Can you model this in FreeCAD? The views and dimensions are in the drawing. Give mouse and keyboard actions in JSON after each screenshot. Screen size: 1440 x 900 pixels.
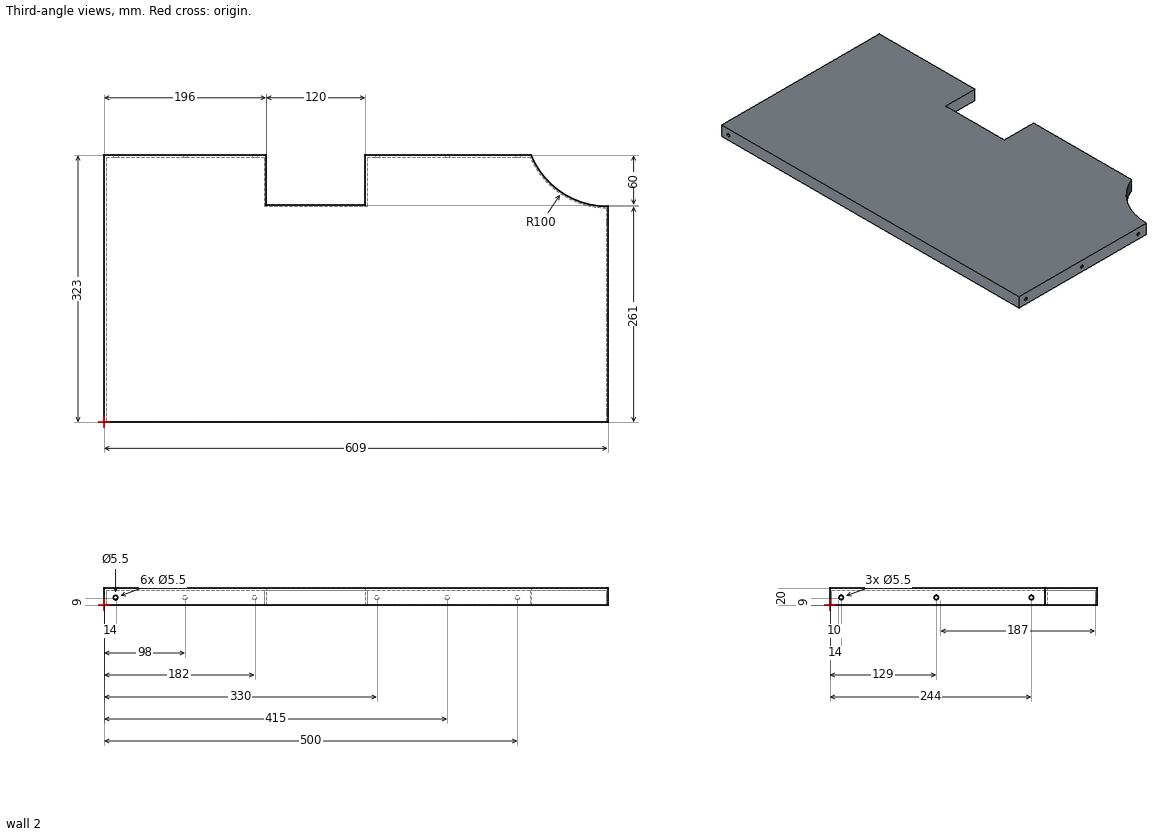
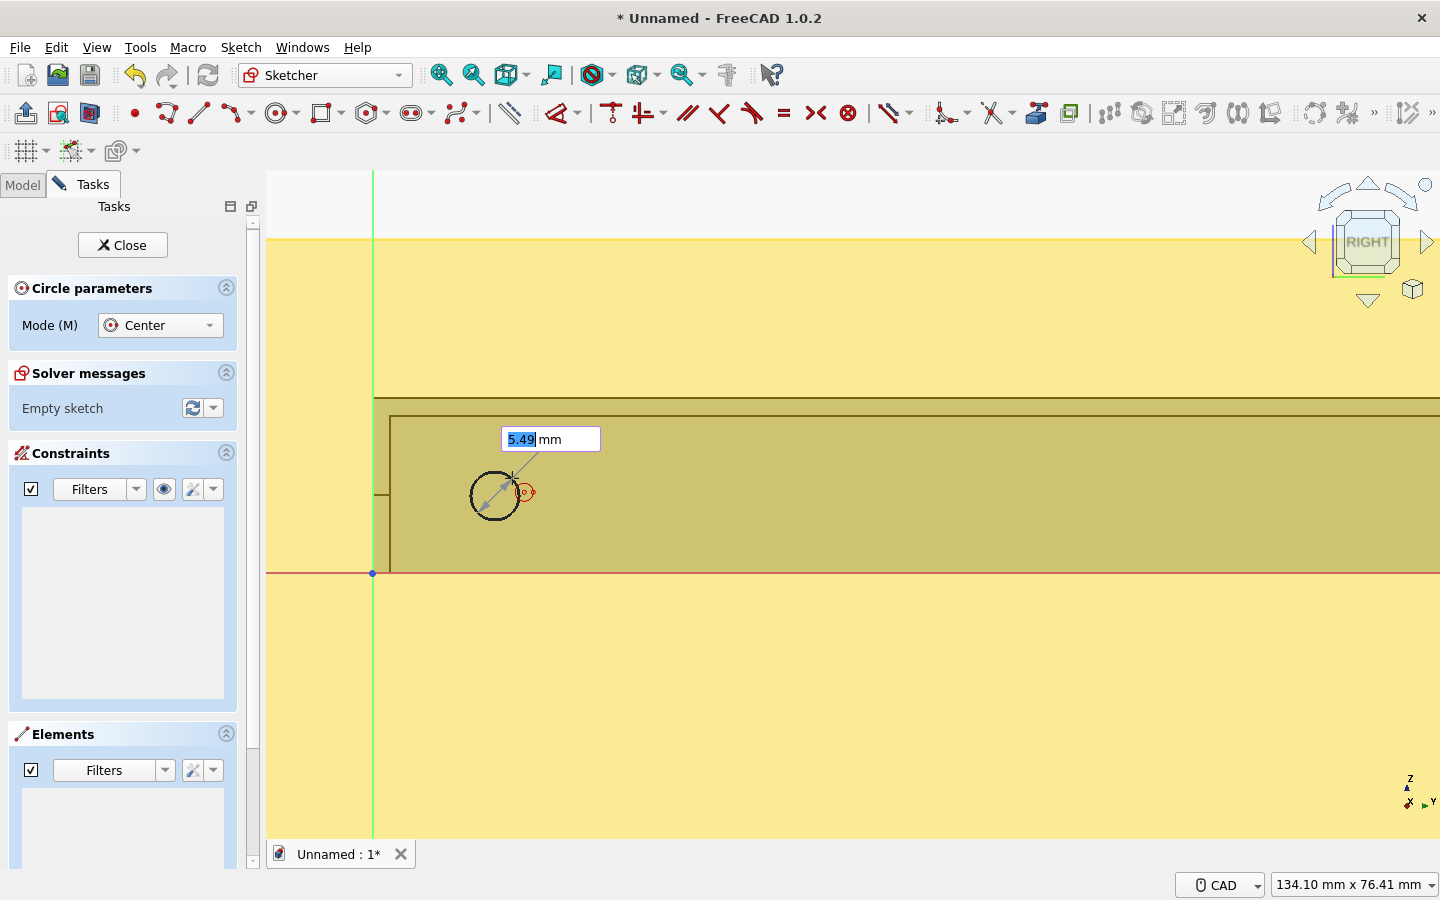
{"action": "type", "text": "5.5"}
{"action": "key", "text": "Return"}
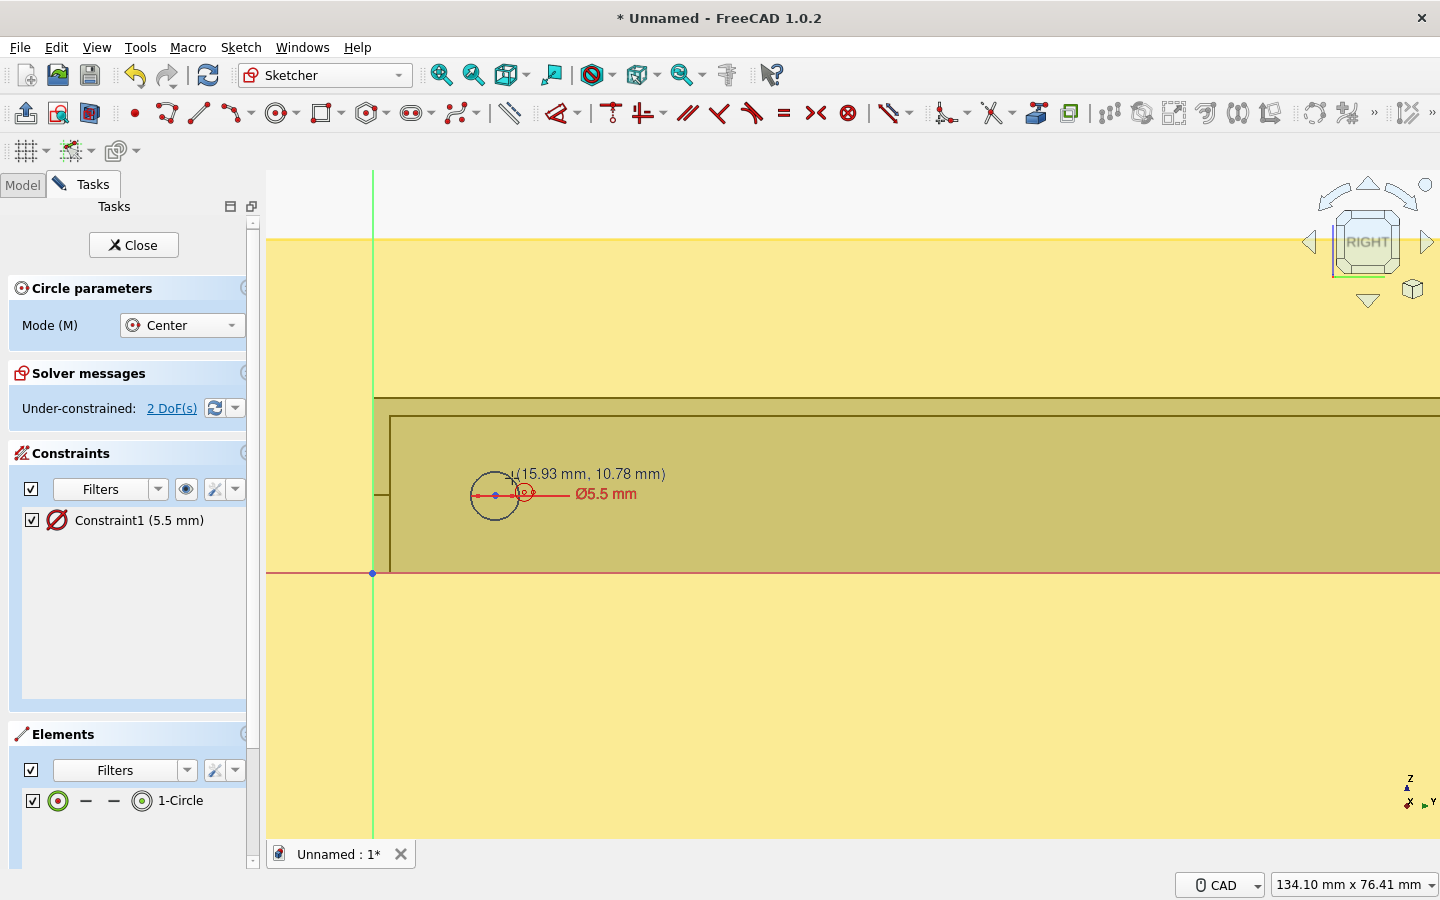
{"action": "scroll", "coordinate": [497, 497], "scroll_direction": "down", "scroll_amount": 6}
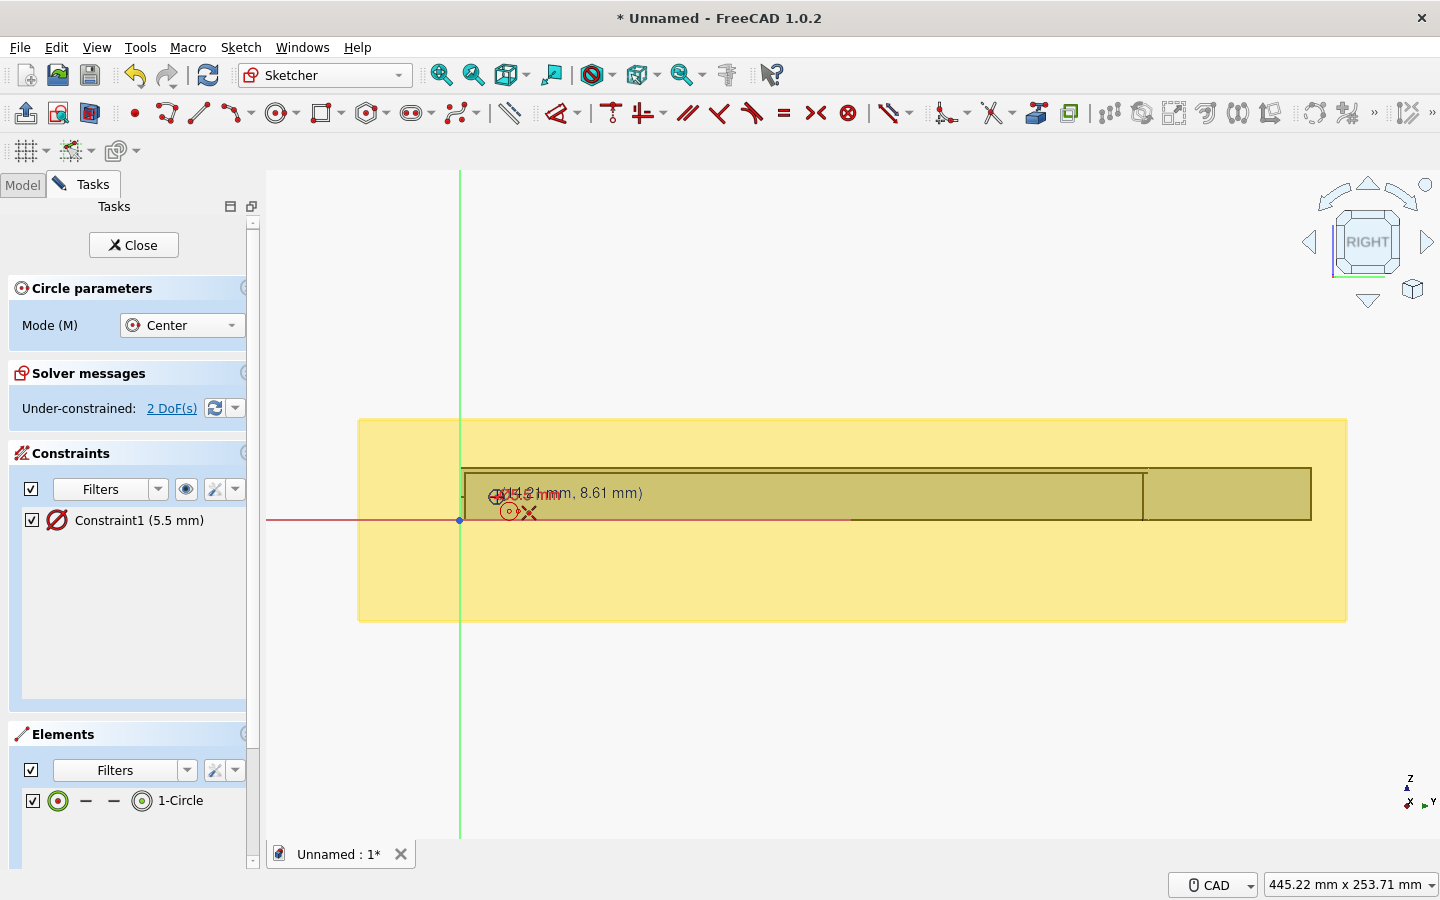
{"action": "scroll", "coordinate": [800, 497], "scroll_direction": "up", "scroll_amount": 6}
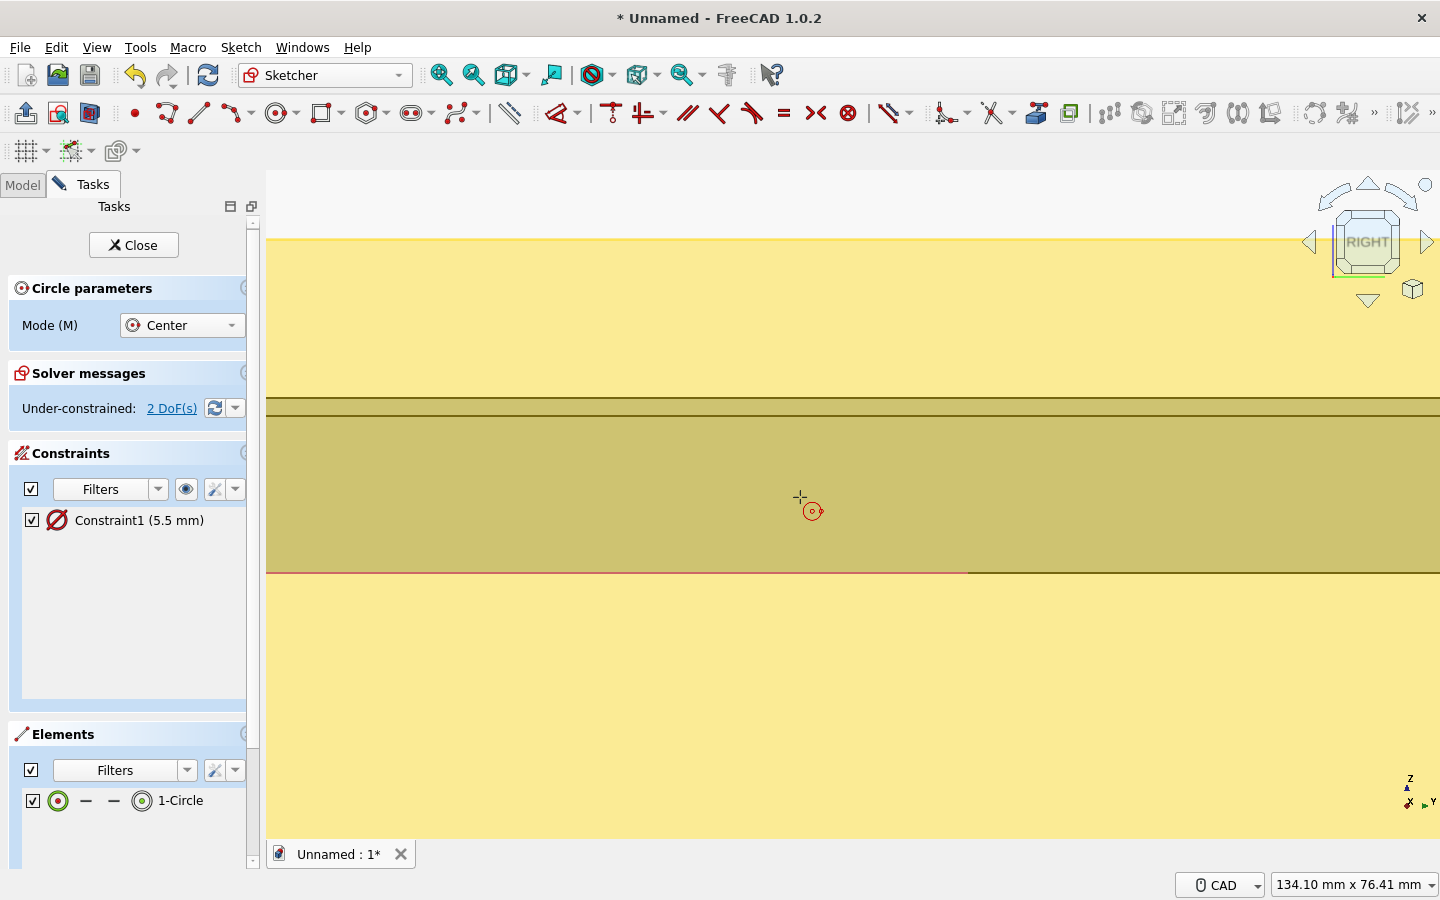
{"action": "left_click", "coordinate": [798, 495]}
{"action": "mouse_move", "coordinate": [815, 478]}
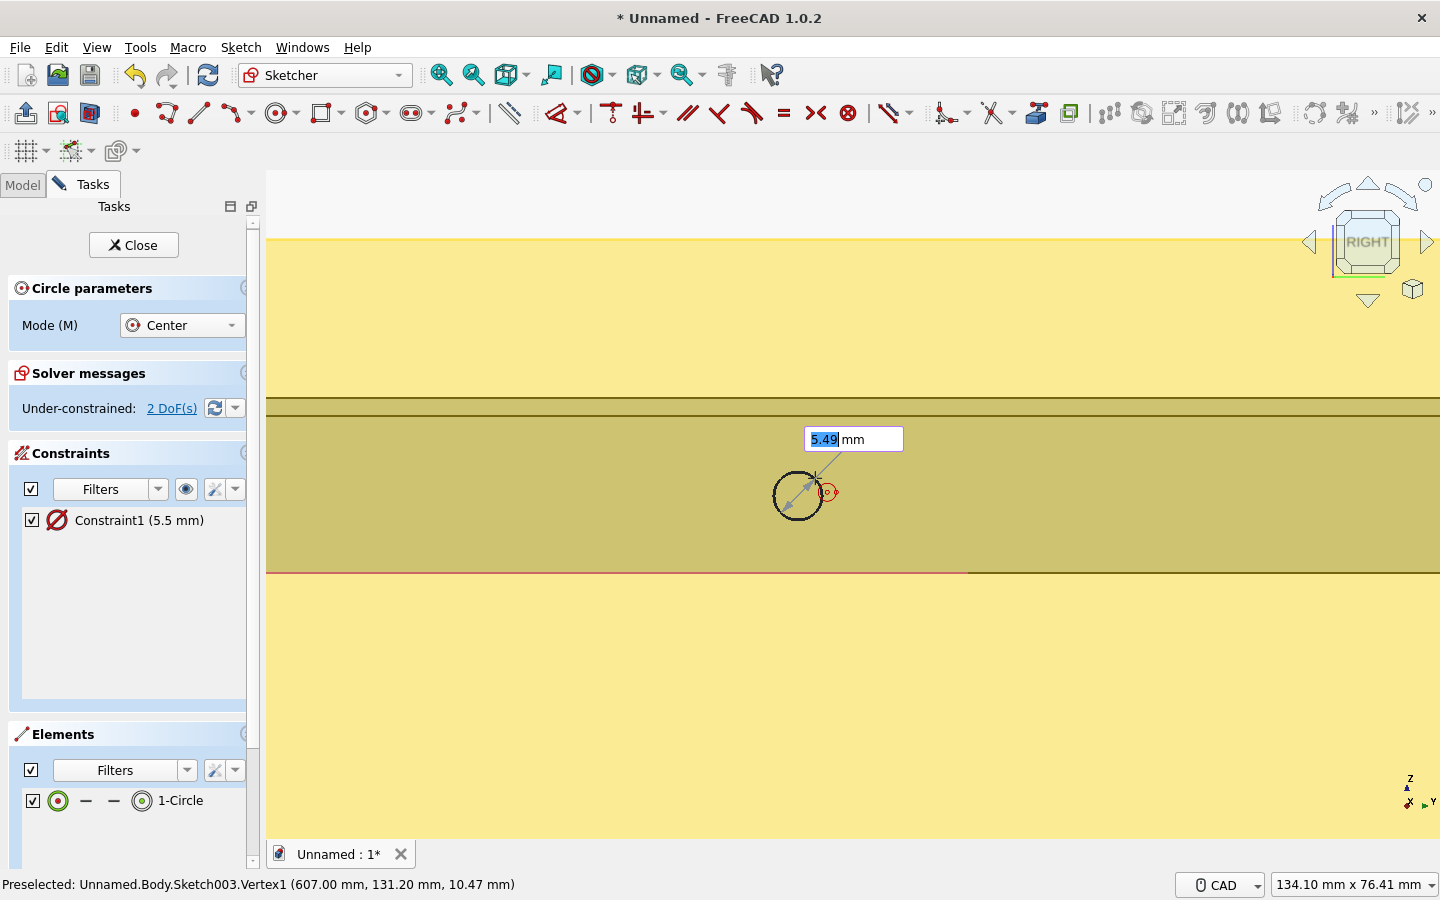
{"action": "type", "text": "5.5"}
{"action": "key", "text": "Return"}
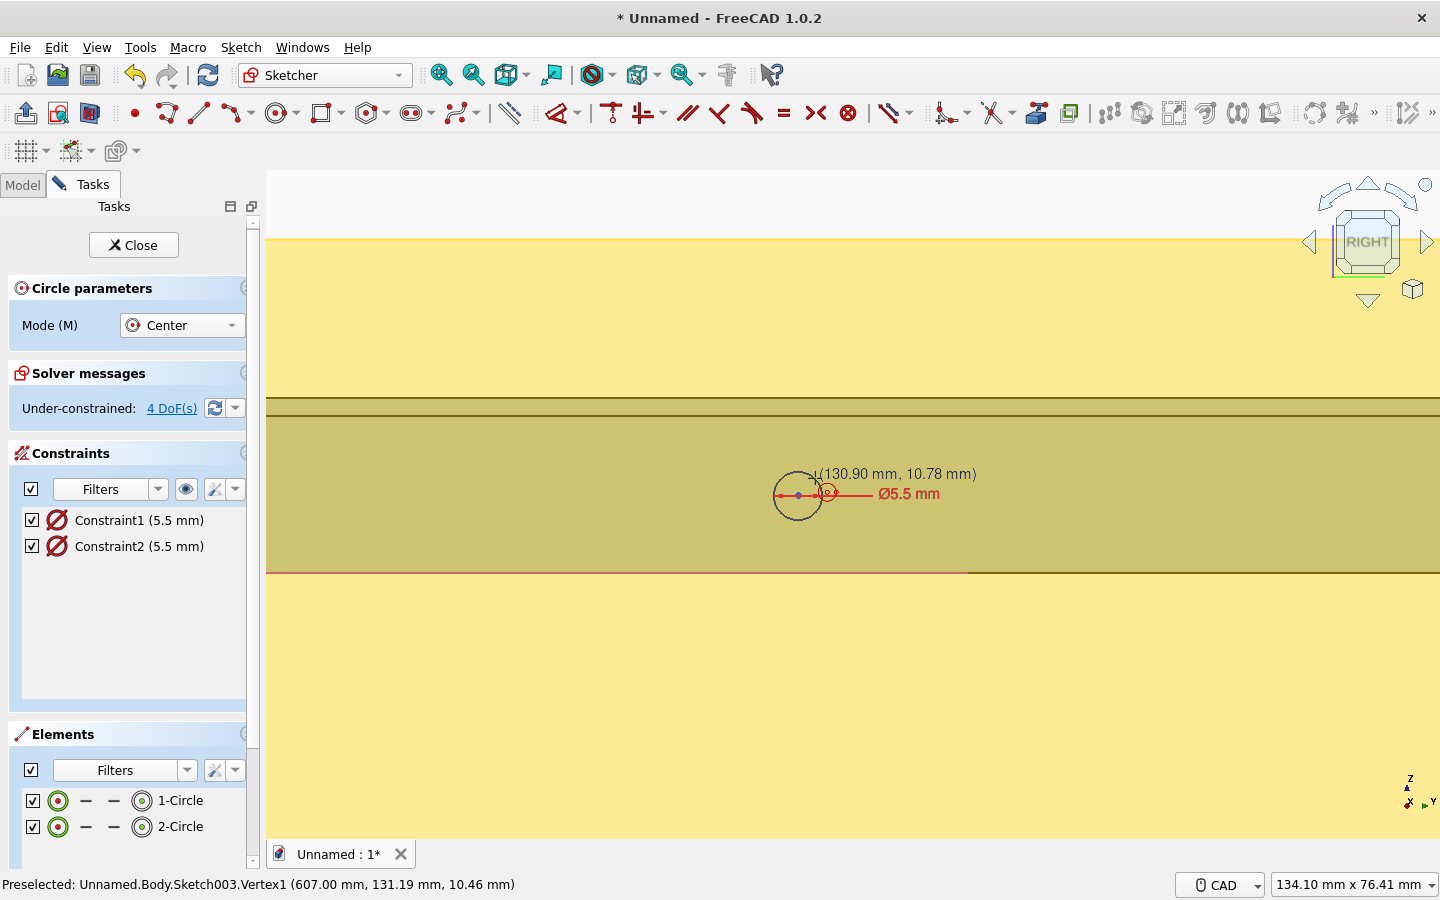
{"action": "scroll", "coordinate": [800, 497], "scroll_direction": "down", "scroll_amount": 6}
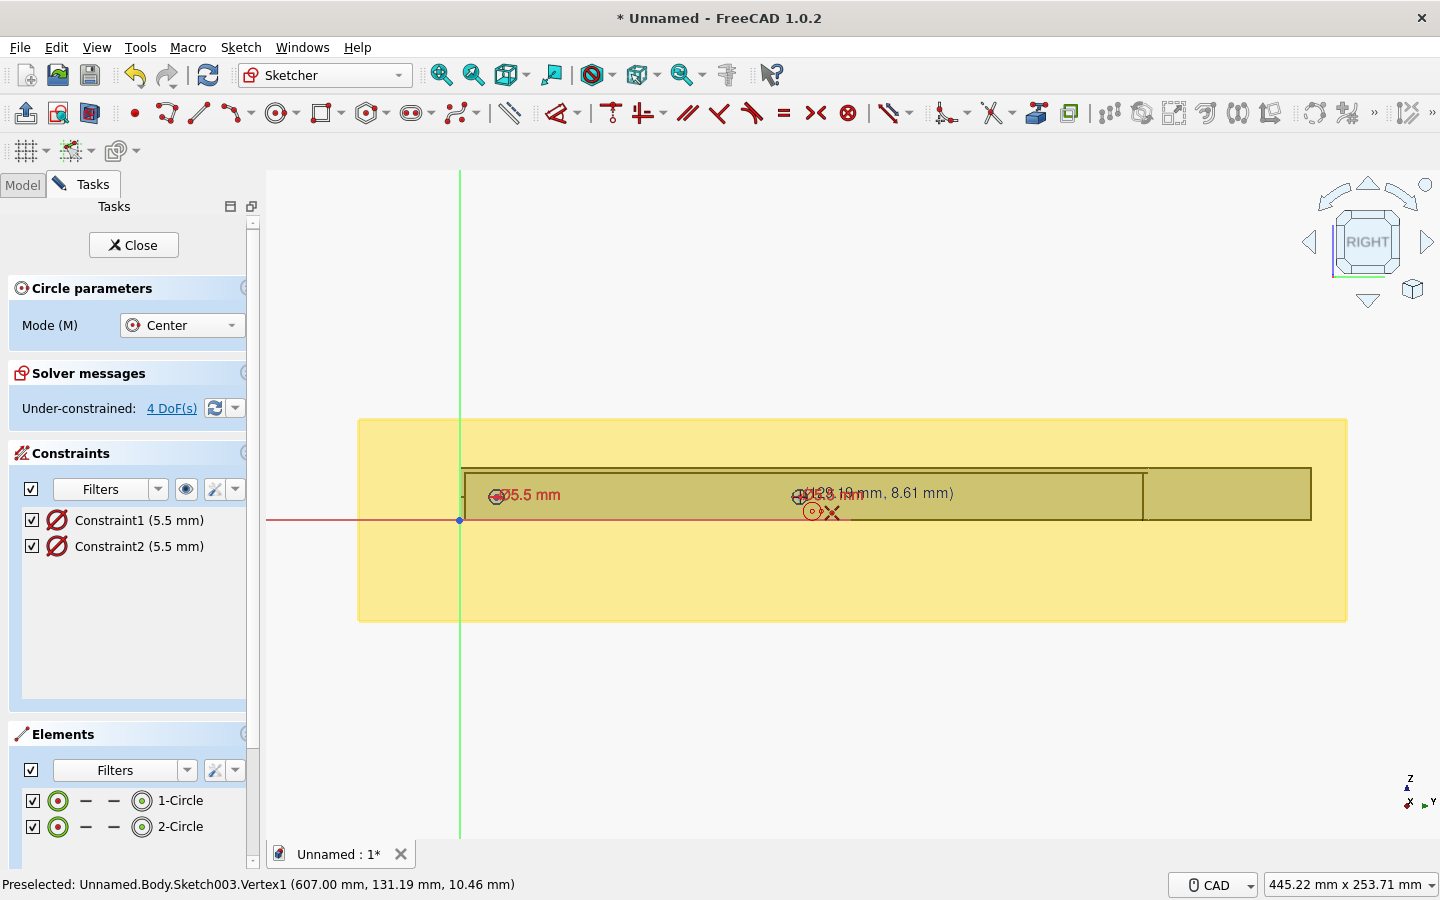
{"action": "scroll", "coordinate": [1103, 497], "scroll_direction": "up", "scroll_amount": 6}